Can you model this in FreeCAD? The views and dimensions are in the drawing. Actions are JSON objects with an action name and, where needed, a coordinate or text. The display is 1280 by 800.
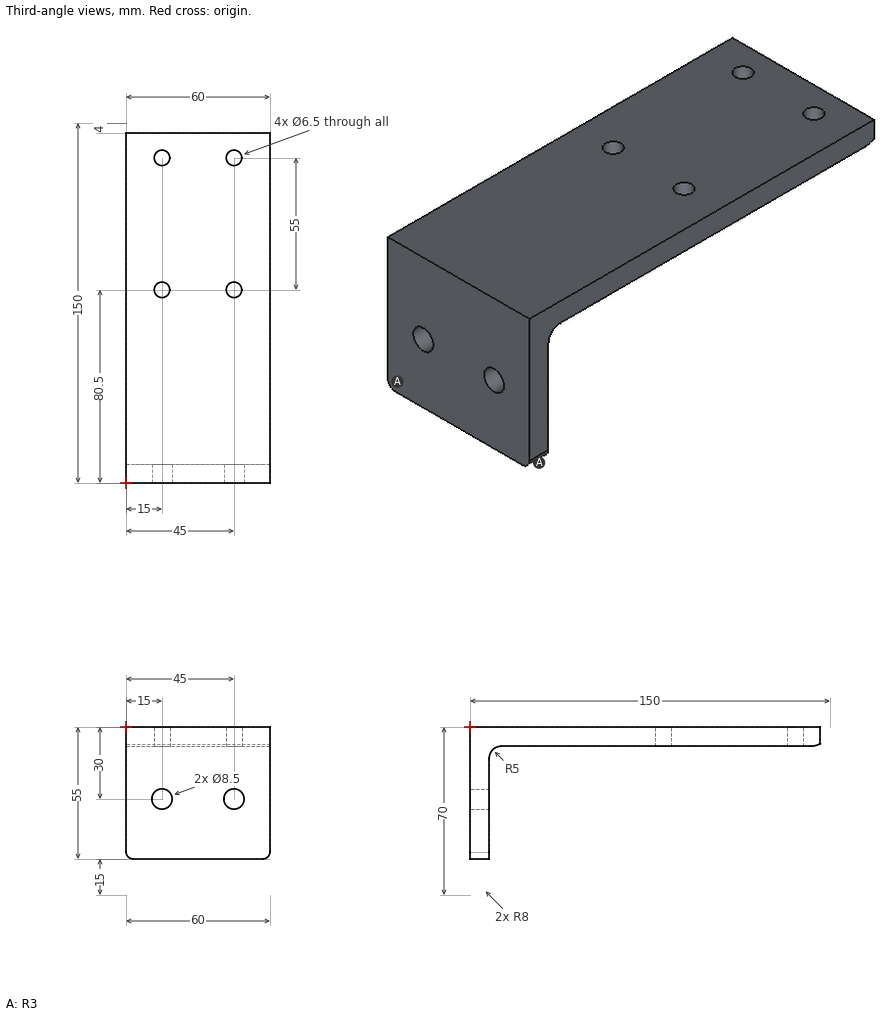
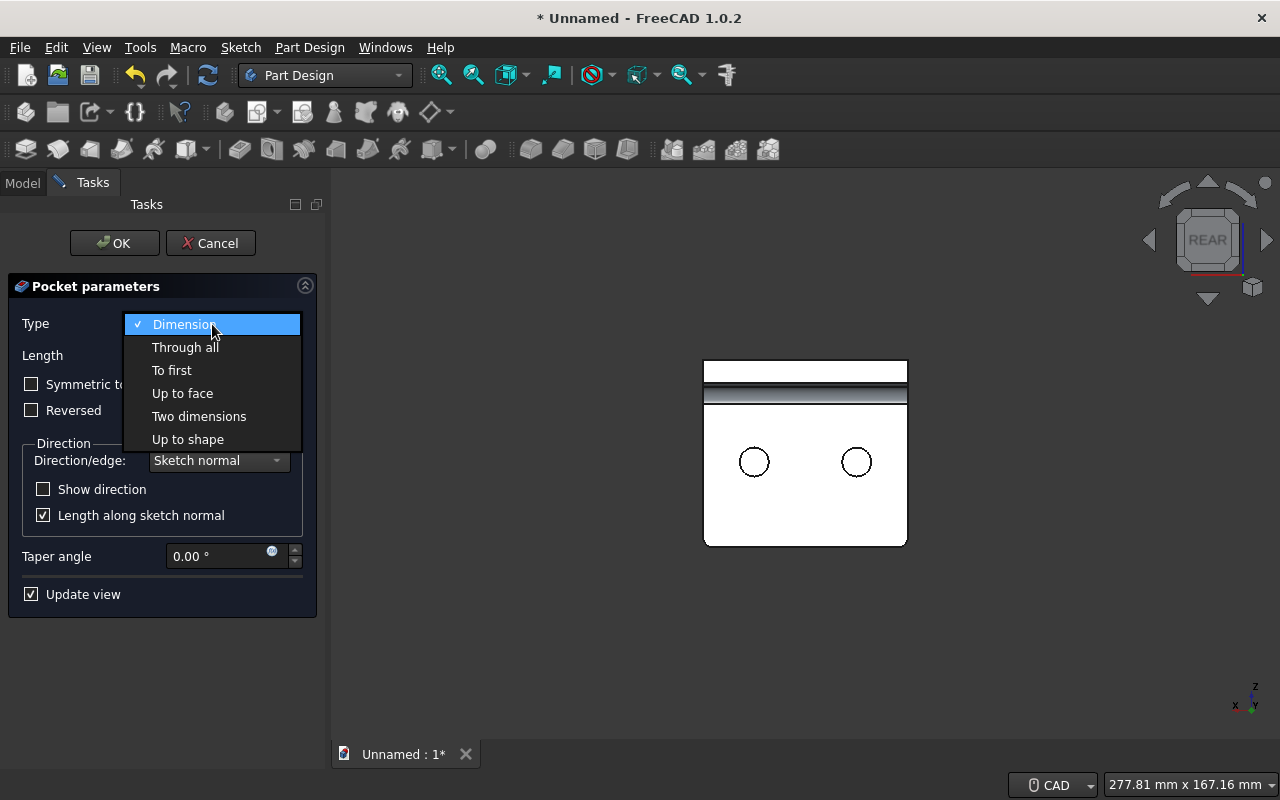
{"action": "left_click", "coordinate": [212, 348]}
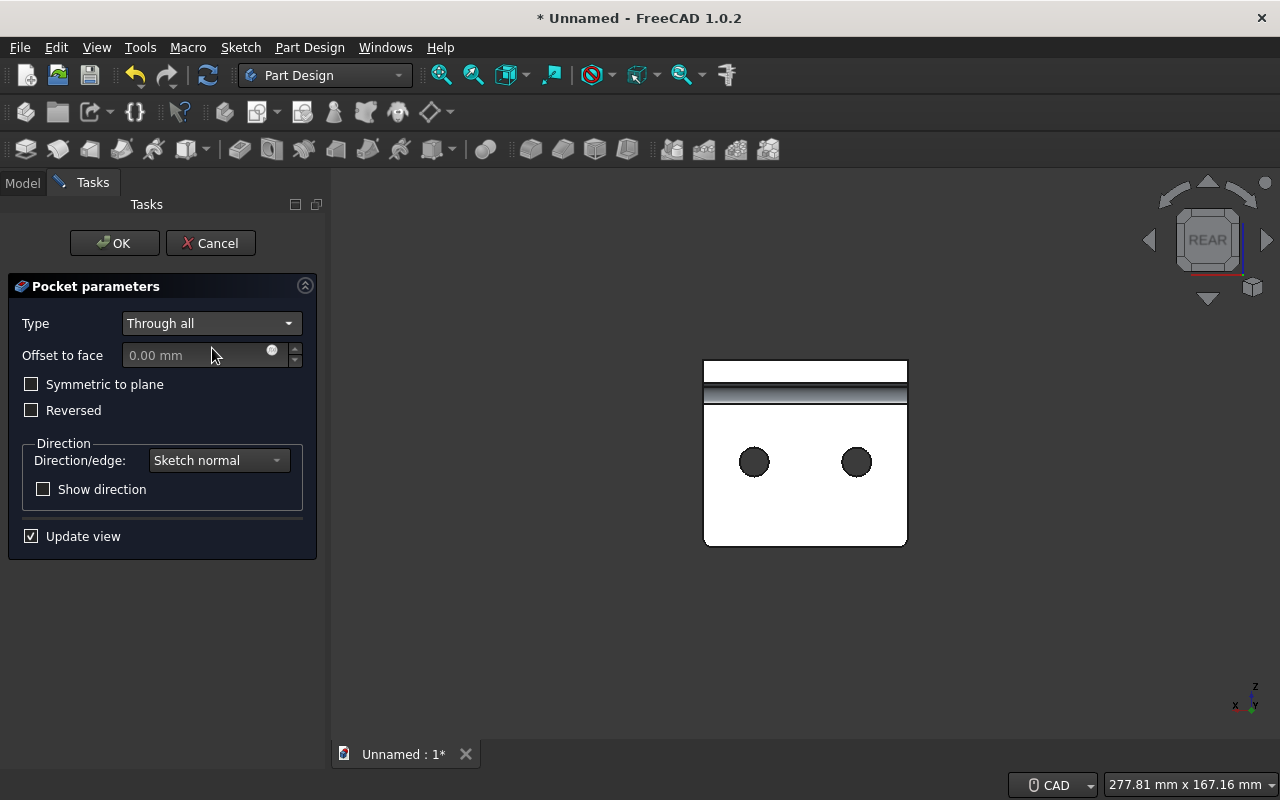
{"action": "left_click", "coordinate": [115, 243]}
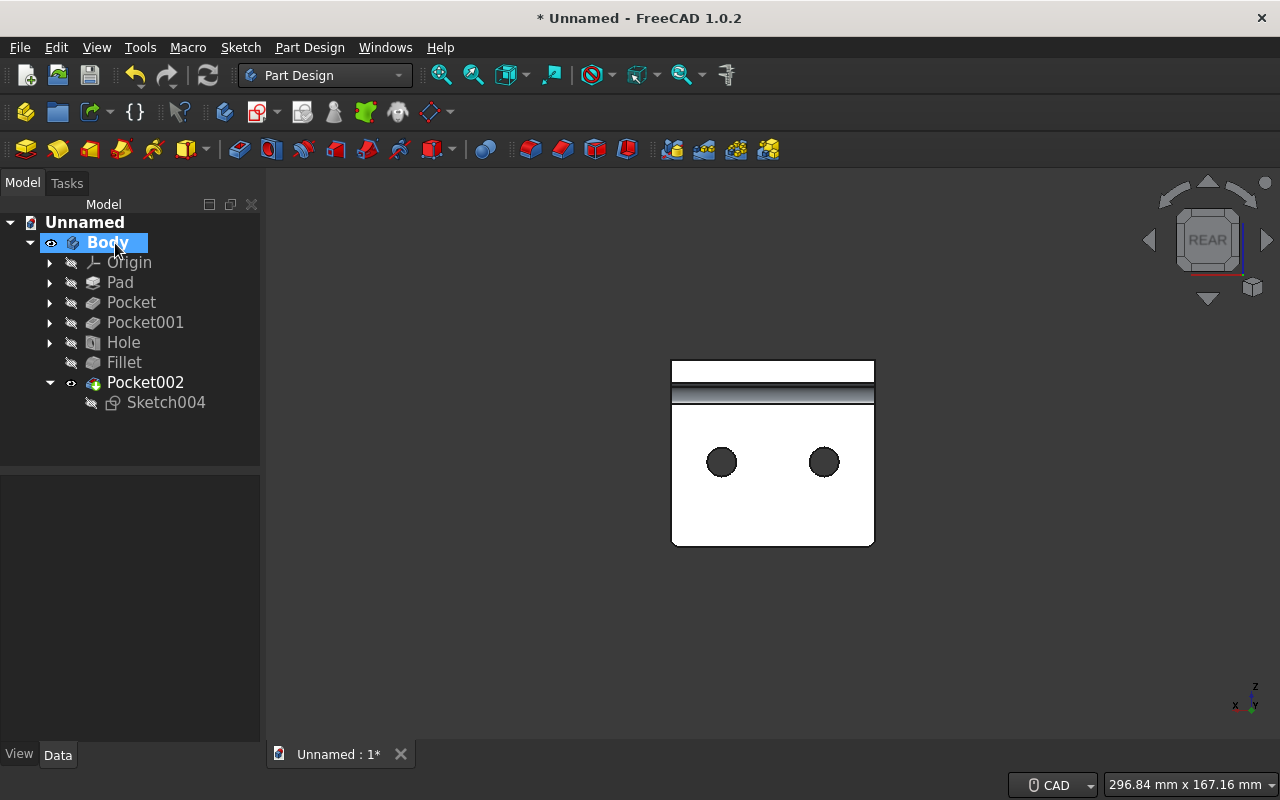
{"action": "key", "text": "0"}